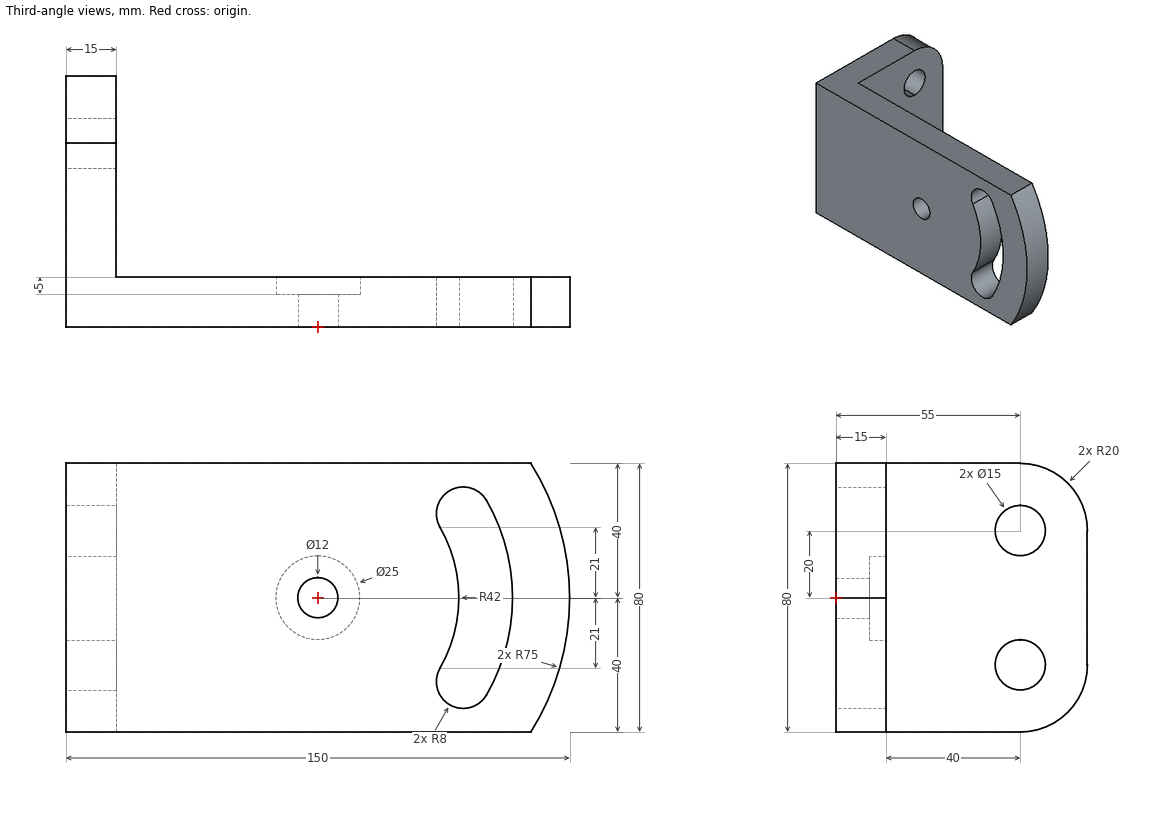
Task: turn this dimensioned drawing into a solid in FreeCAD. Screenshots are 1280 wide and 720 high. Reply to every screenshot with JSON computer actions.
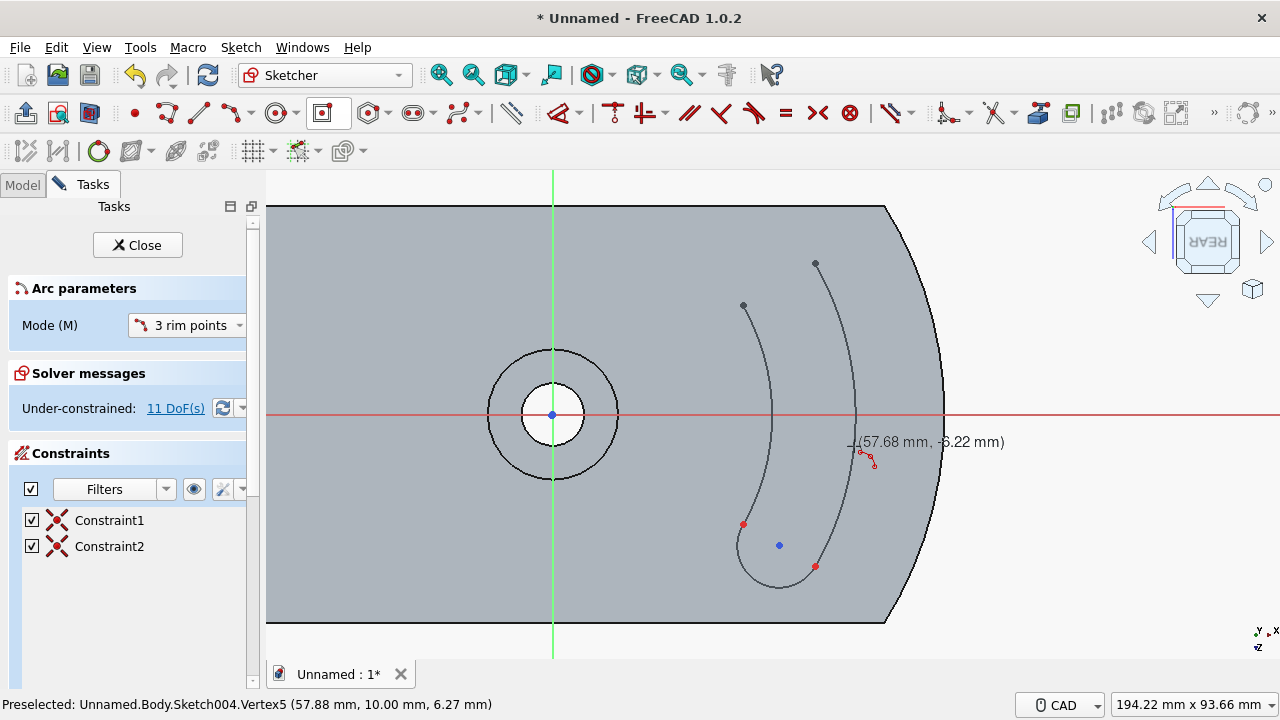
{"action": "left_click", "coordinate": [815, 264]}
{"action": "left_click", "coordinate": [743, 306]}
{"action": "left_click", "coordinate": [758, 248]}
{"action": "key", "text": "Escape"}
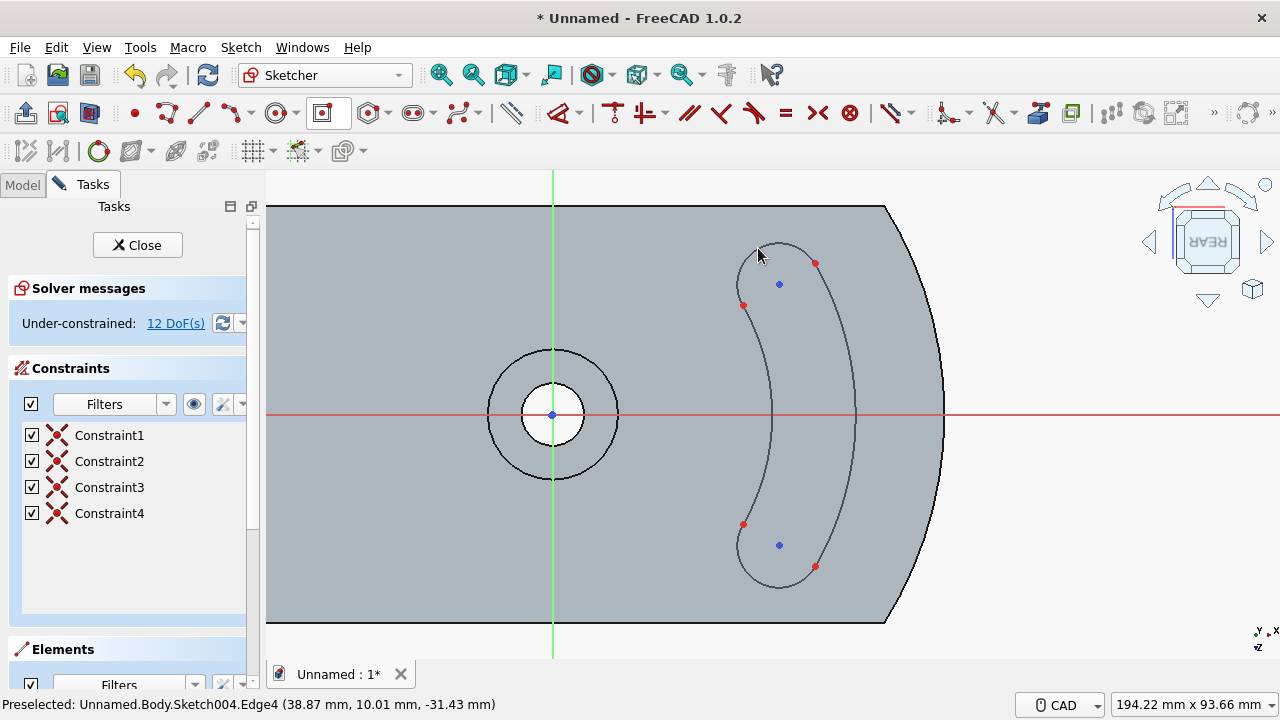
{"action": "left_click", "coordinate": [767, 461]}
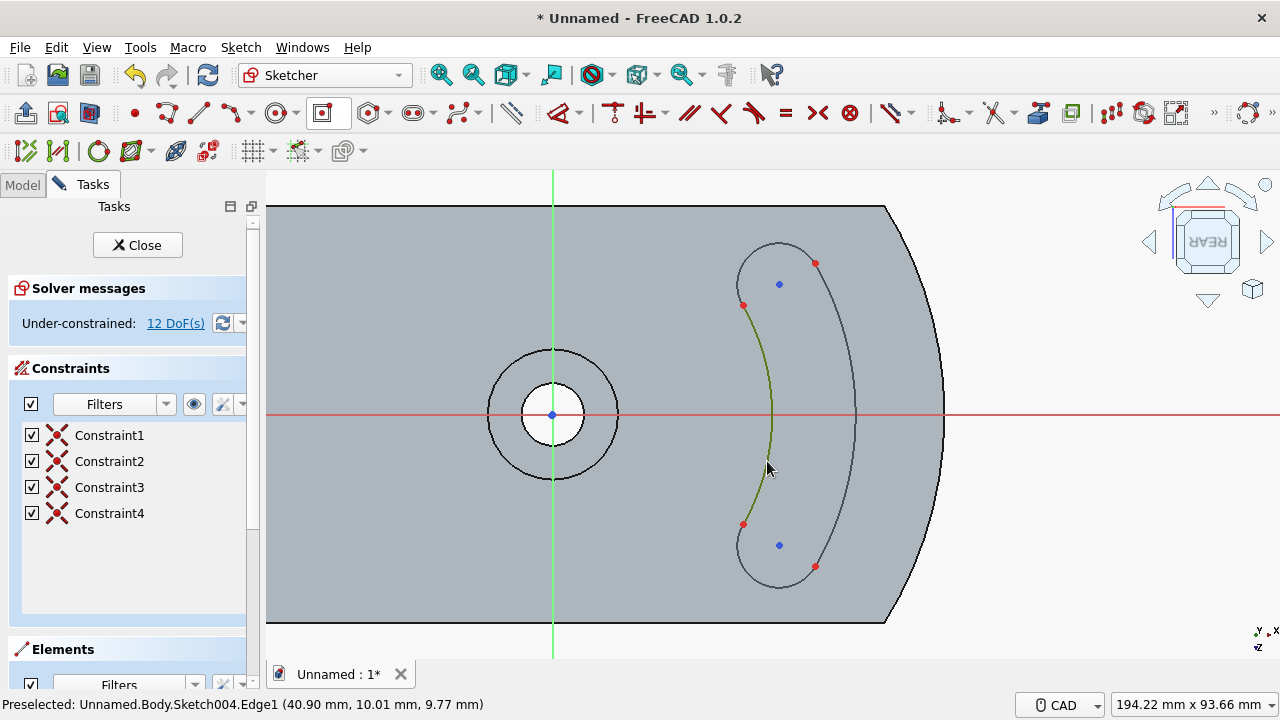
{"action": "left_click", "coordinate": [741, 563]}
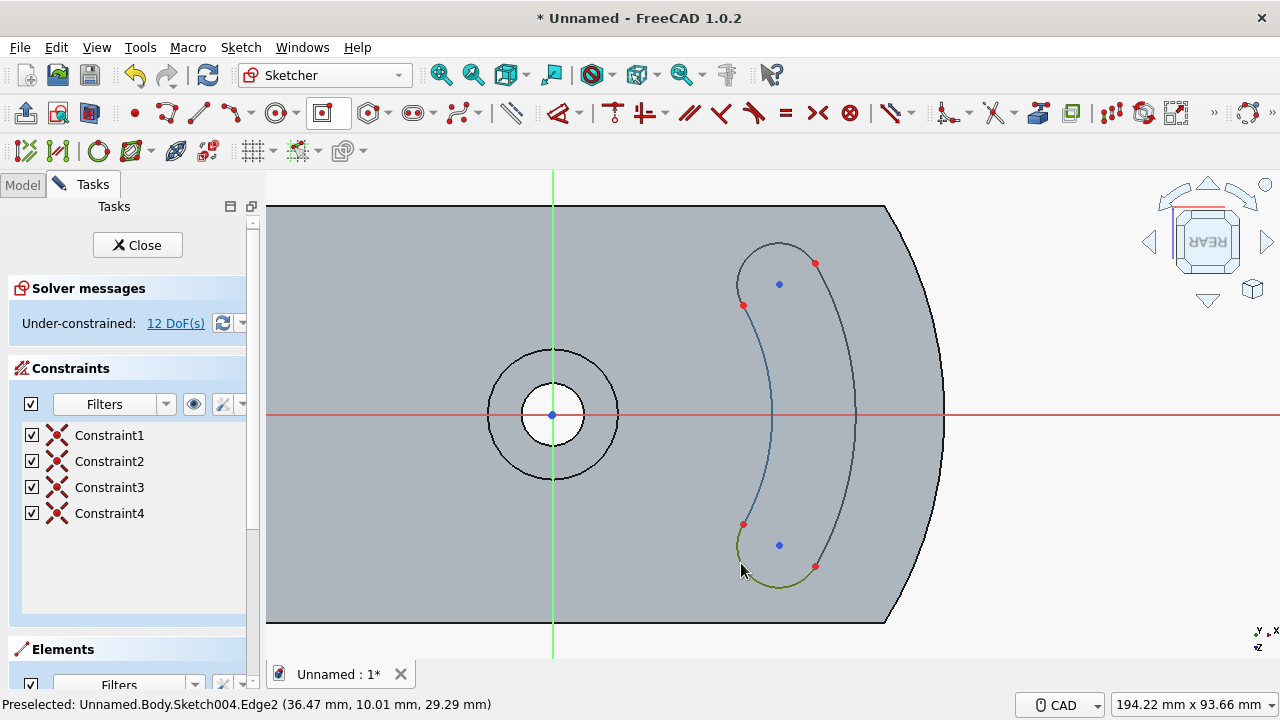
{"action": "left_click", "coordinate": [754, 114]}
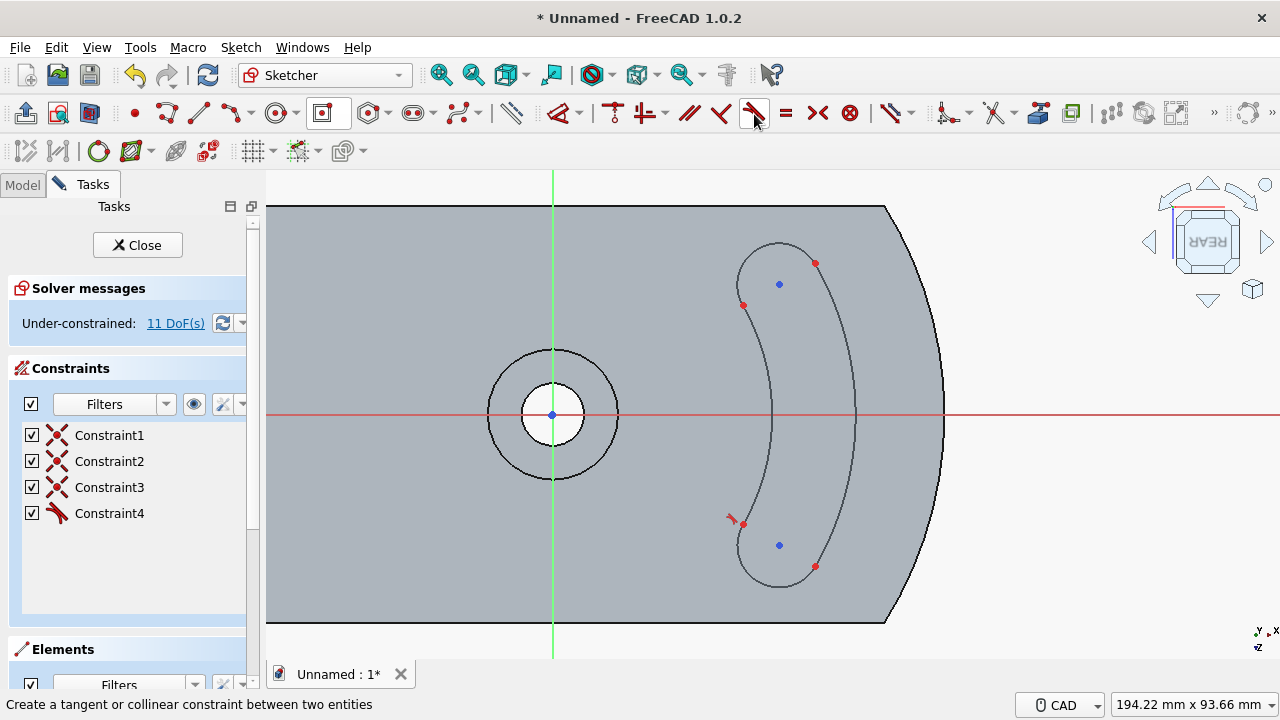
{"action": "left_click", "coordinate": [767, 461]}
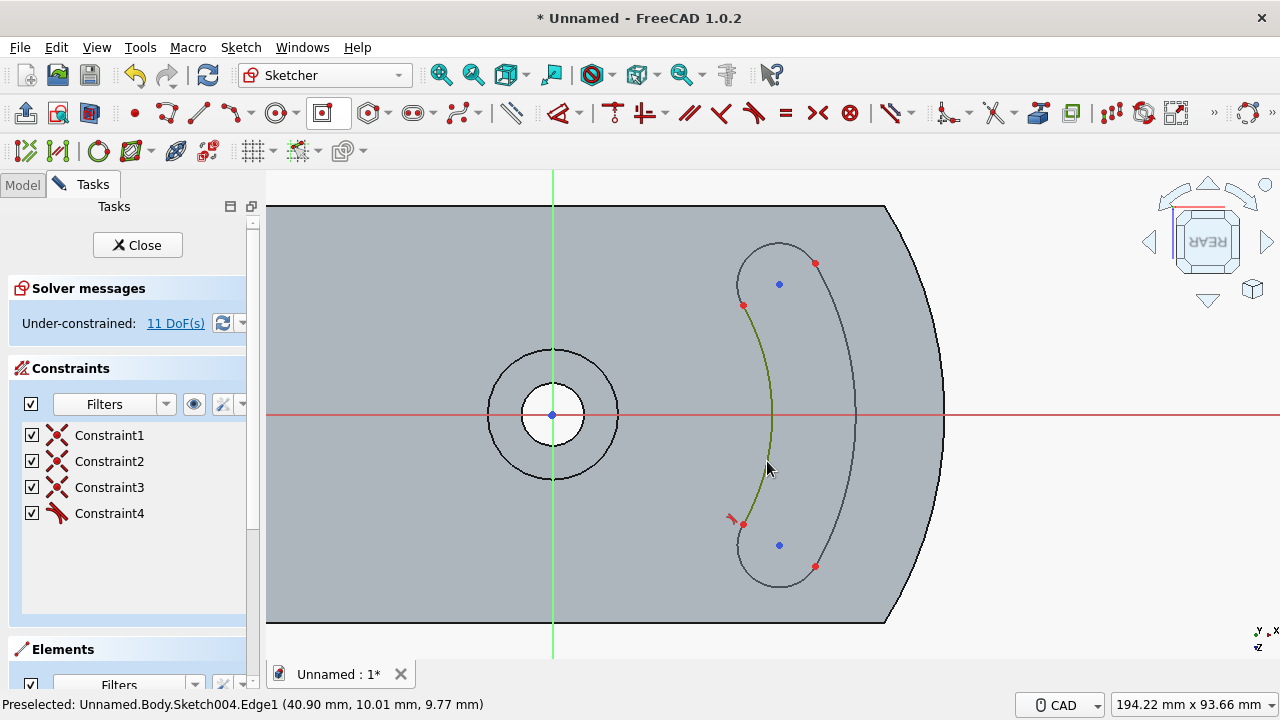
{"action": "left_click", "coordinate": [783, 244]}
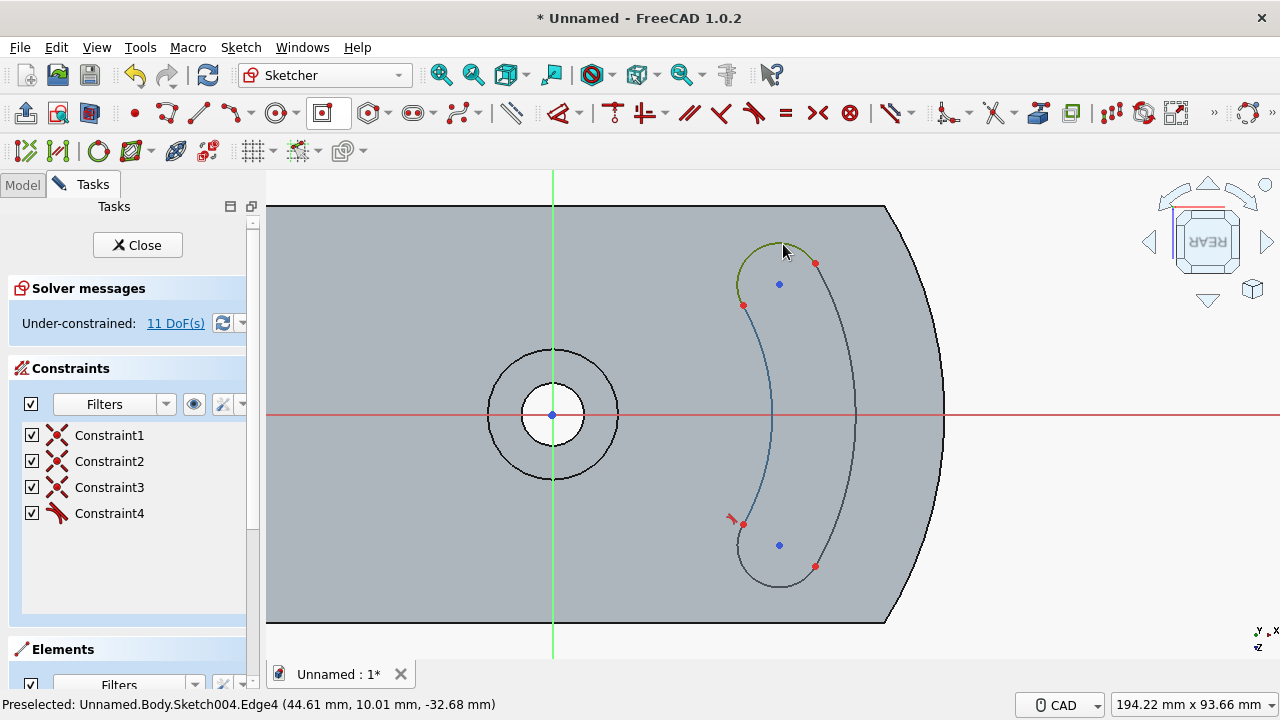
{"action": "key", "text": "t"}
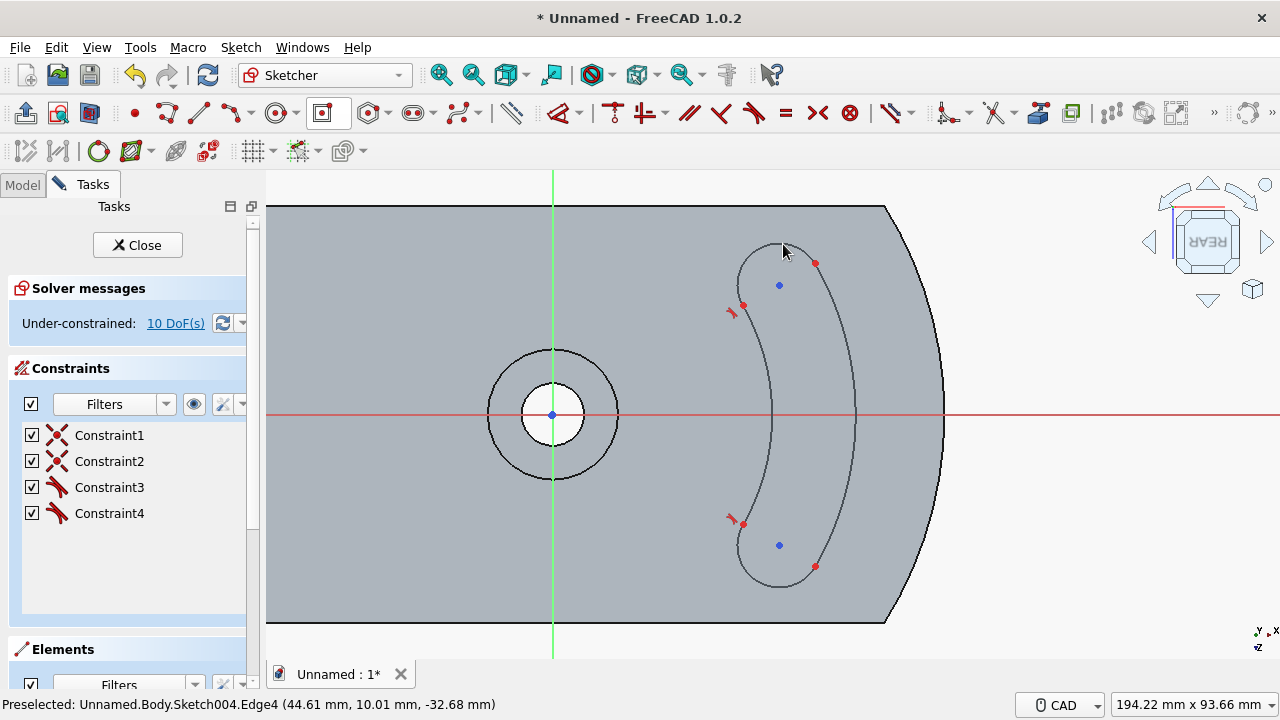
{"action": "left_click", "coordinate": [741, 563]}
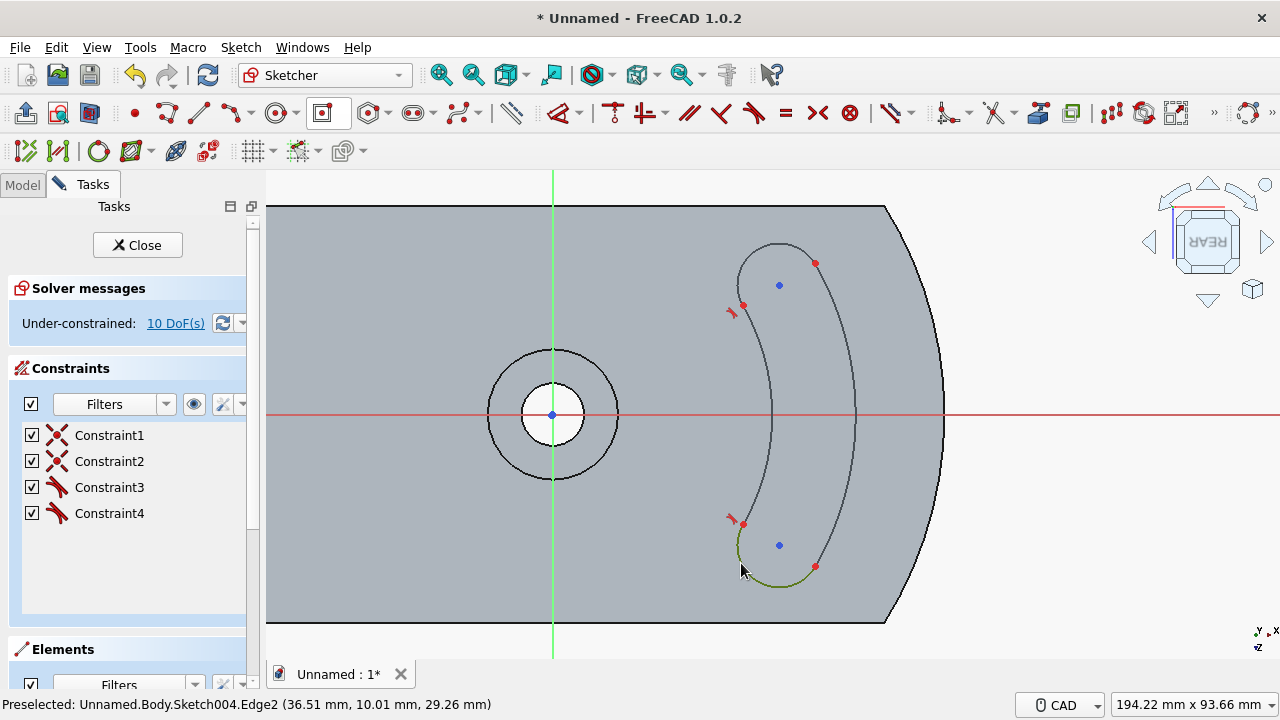
{"action": "left_click", "coordinate": [849, 479]}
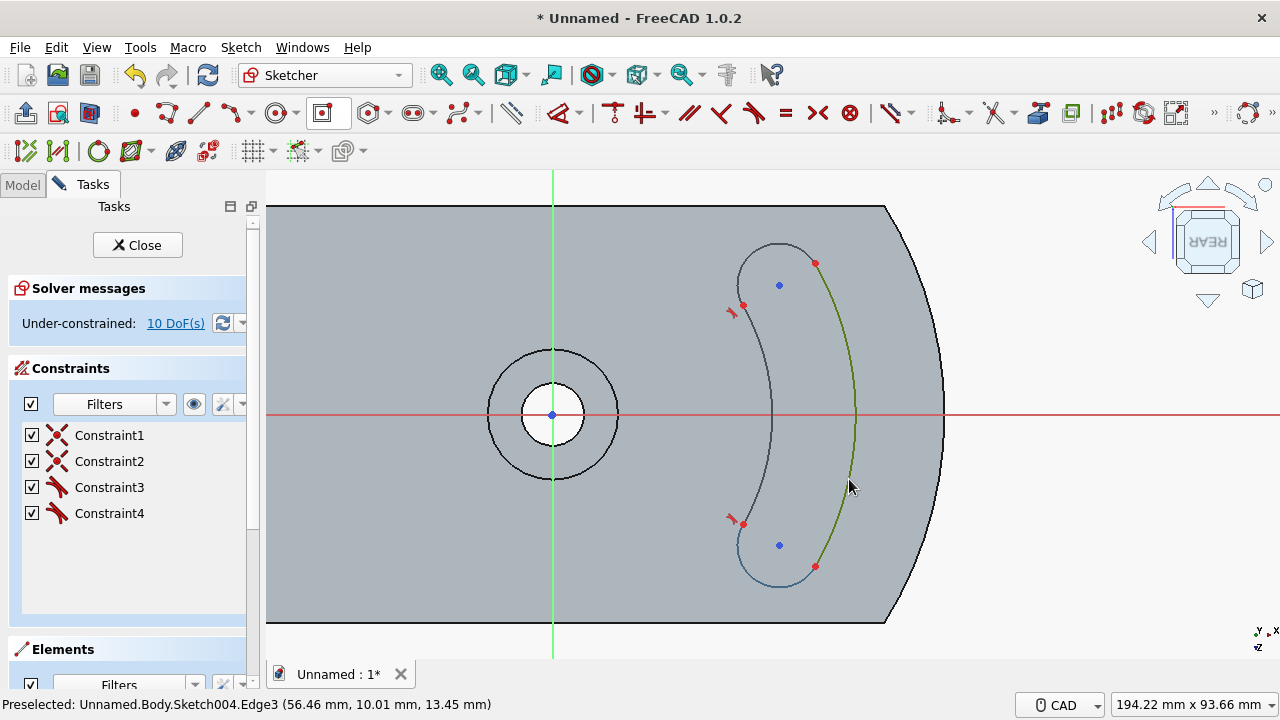
{"action": "left_click", "coordinate": [754, 114]}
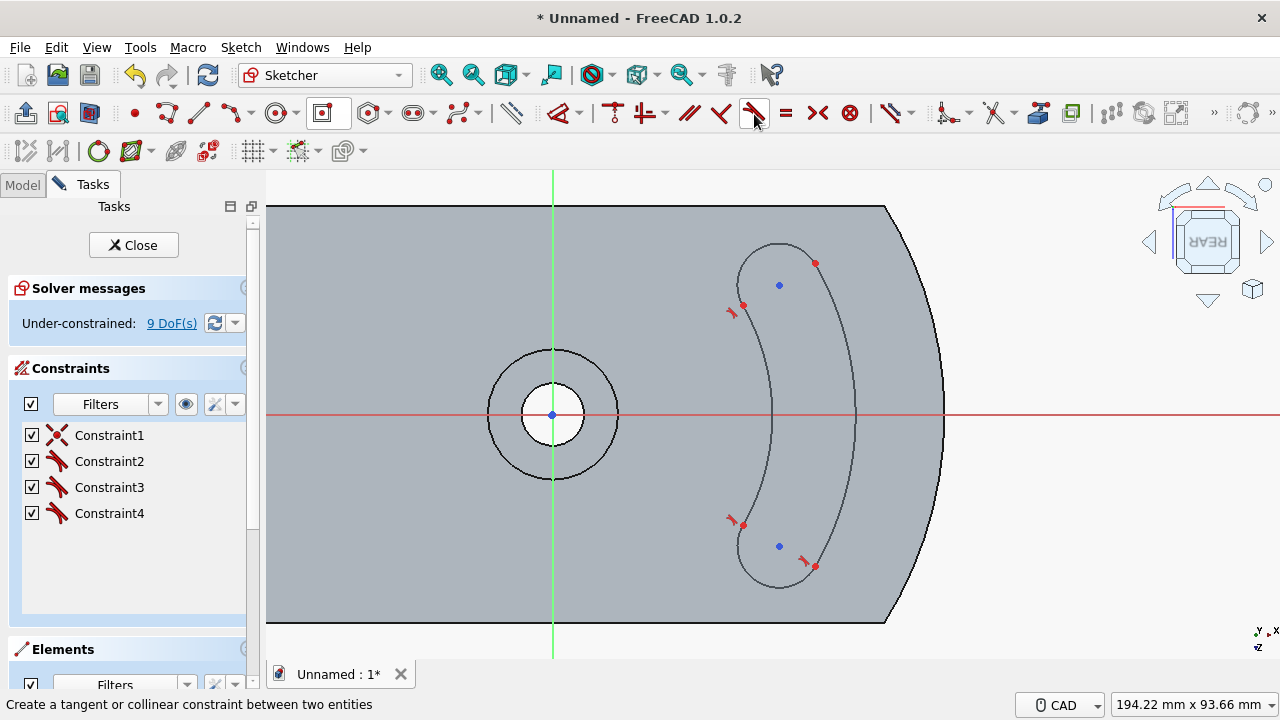
{"action": "left_click", "coordinate": [849, 479]}